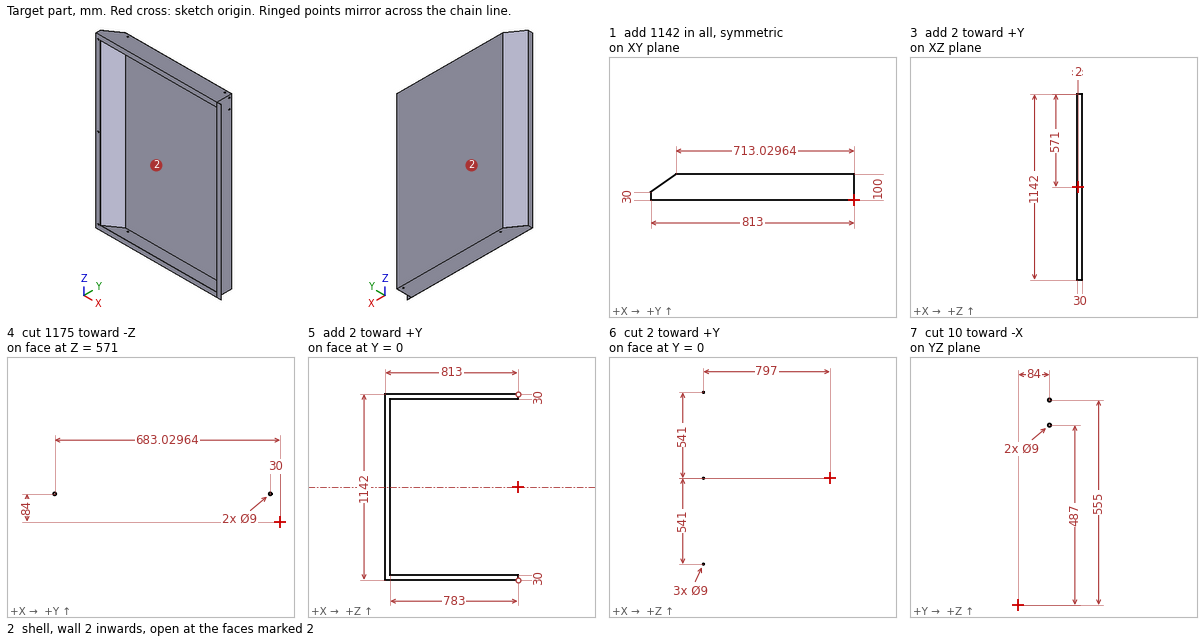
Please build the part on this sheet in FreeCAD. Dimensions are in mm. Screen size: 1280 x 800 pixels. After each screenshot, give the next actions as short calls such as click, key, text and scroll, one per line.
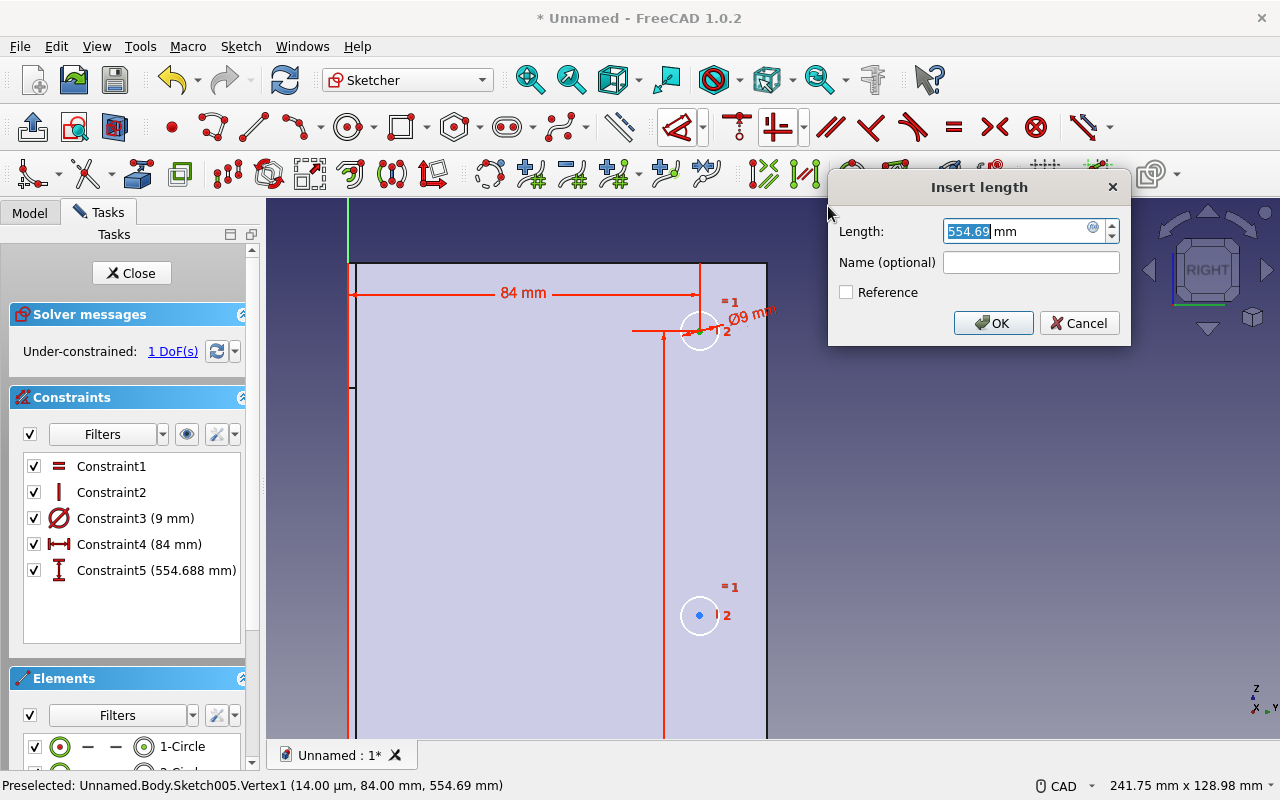
text(555)
key(Return)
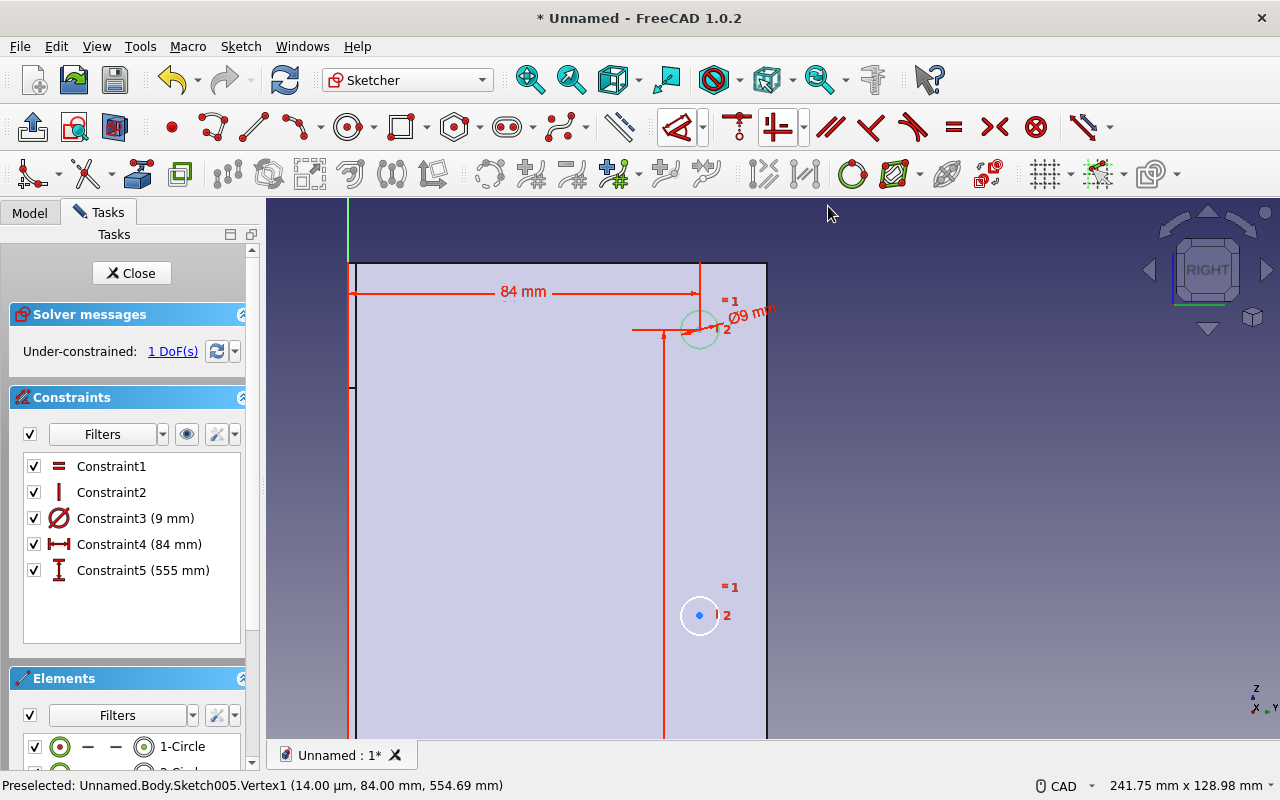
click(700, 616)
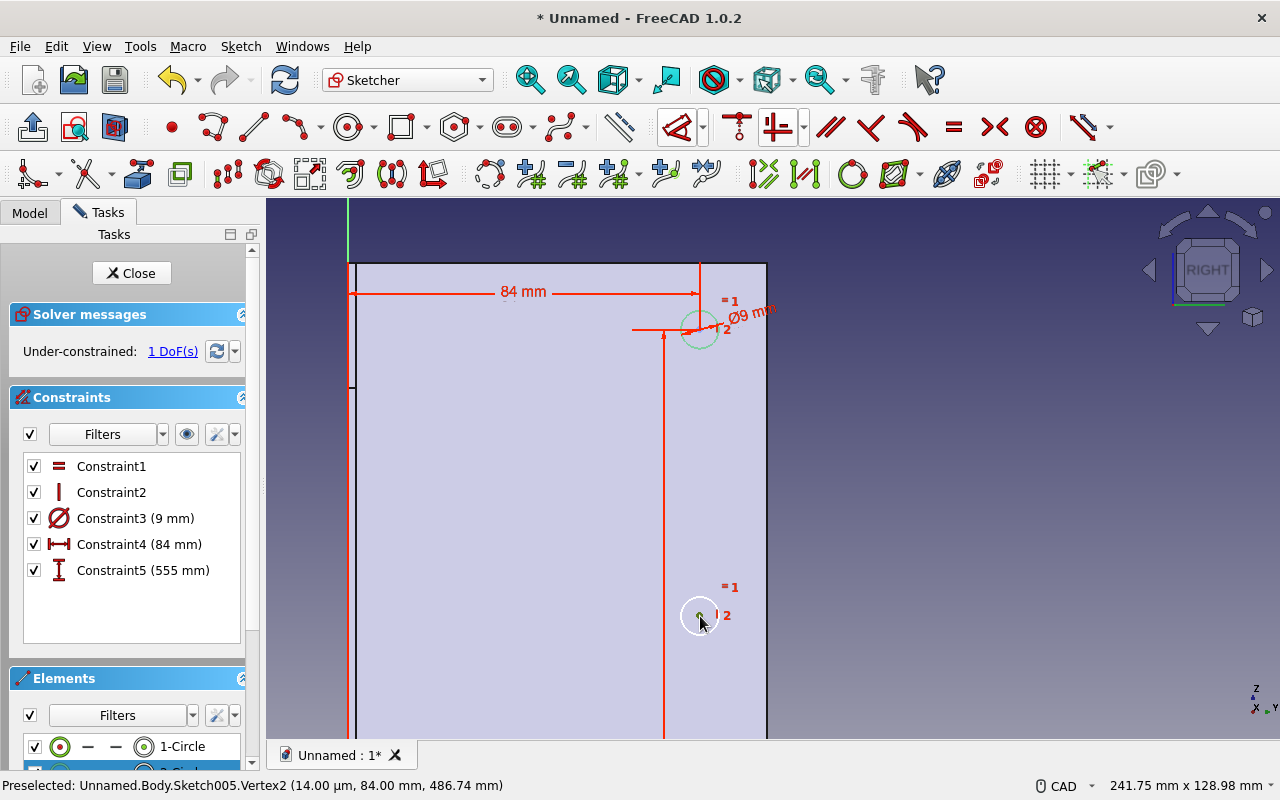
key(i)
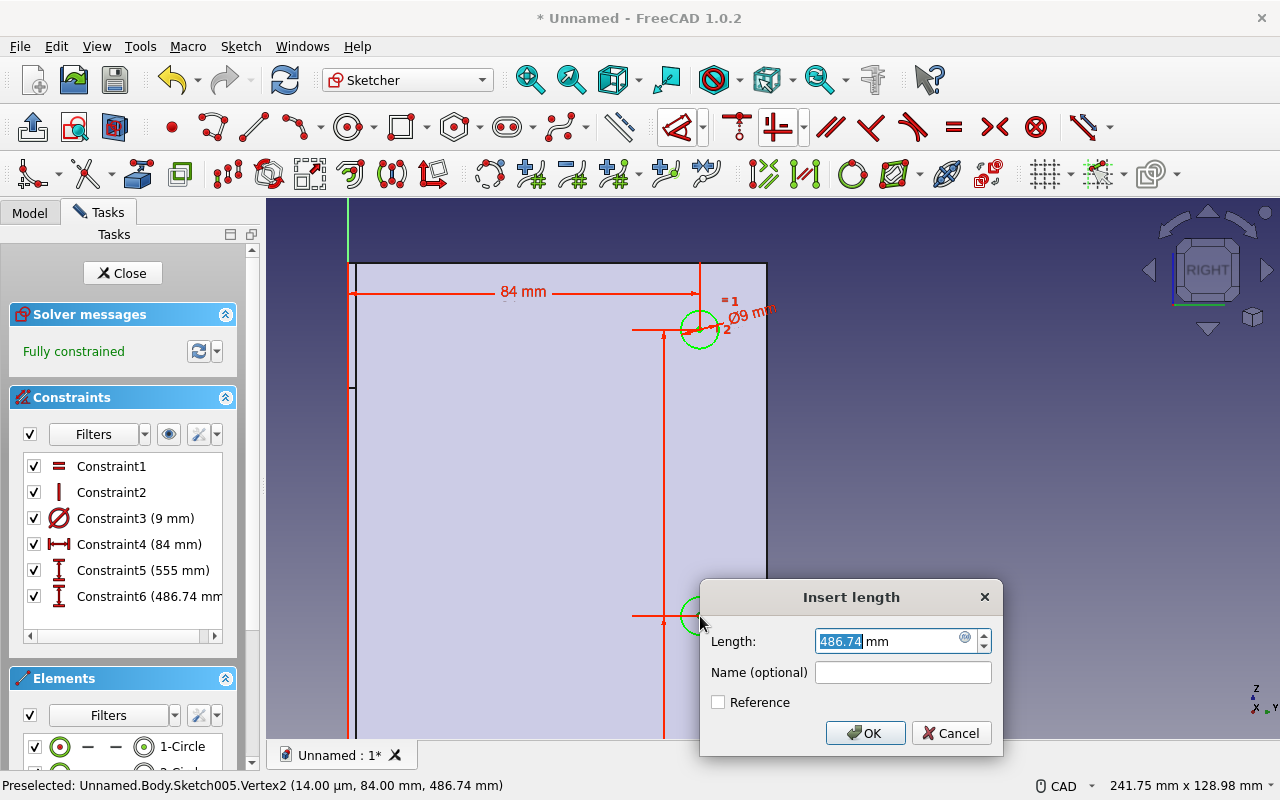
text(487)
key(Return)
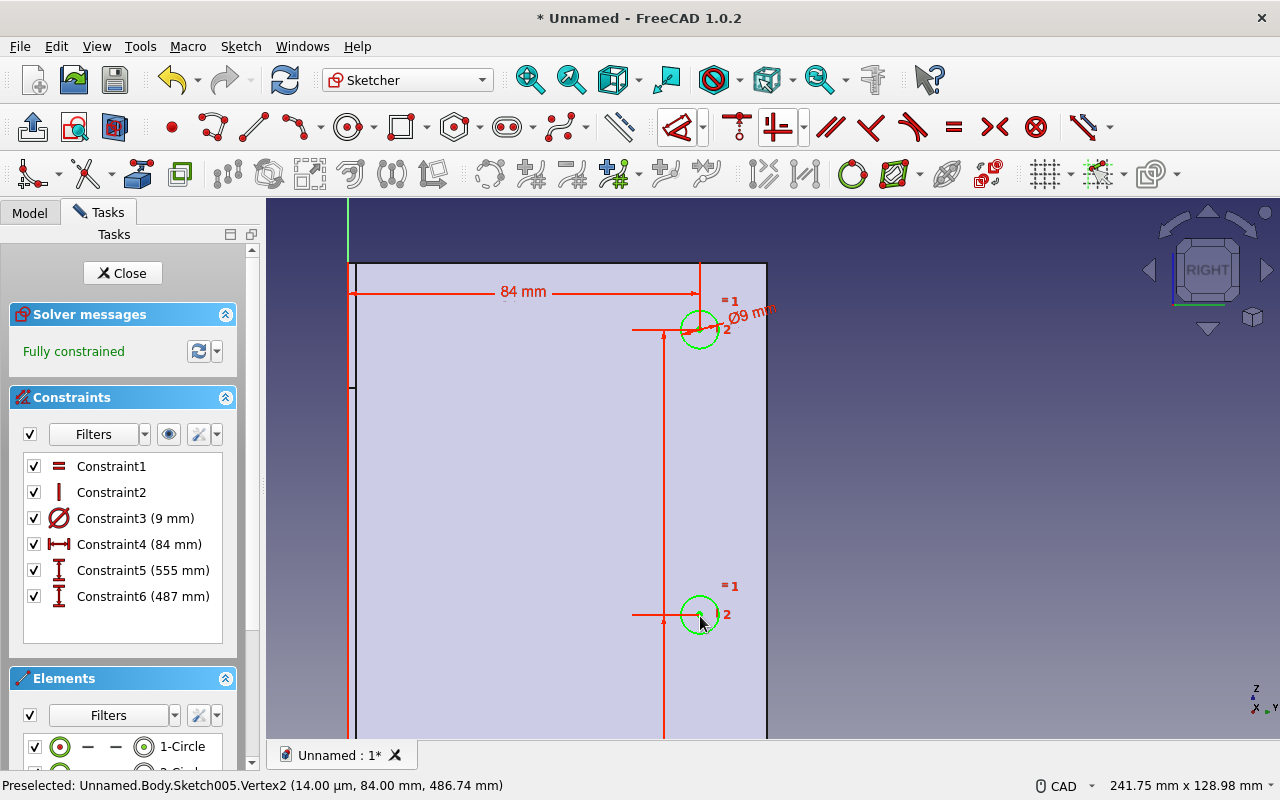
click(123, 273)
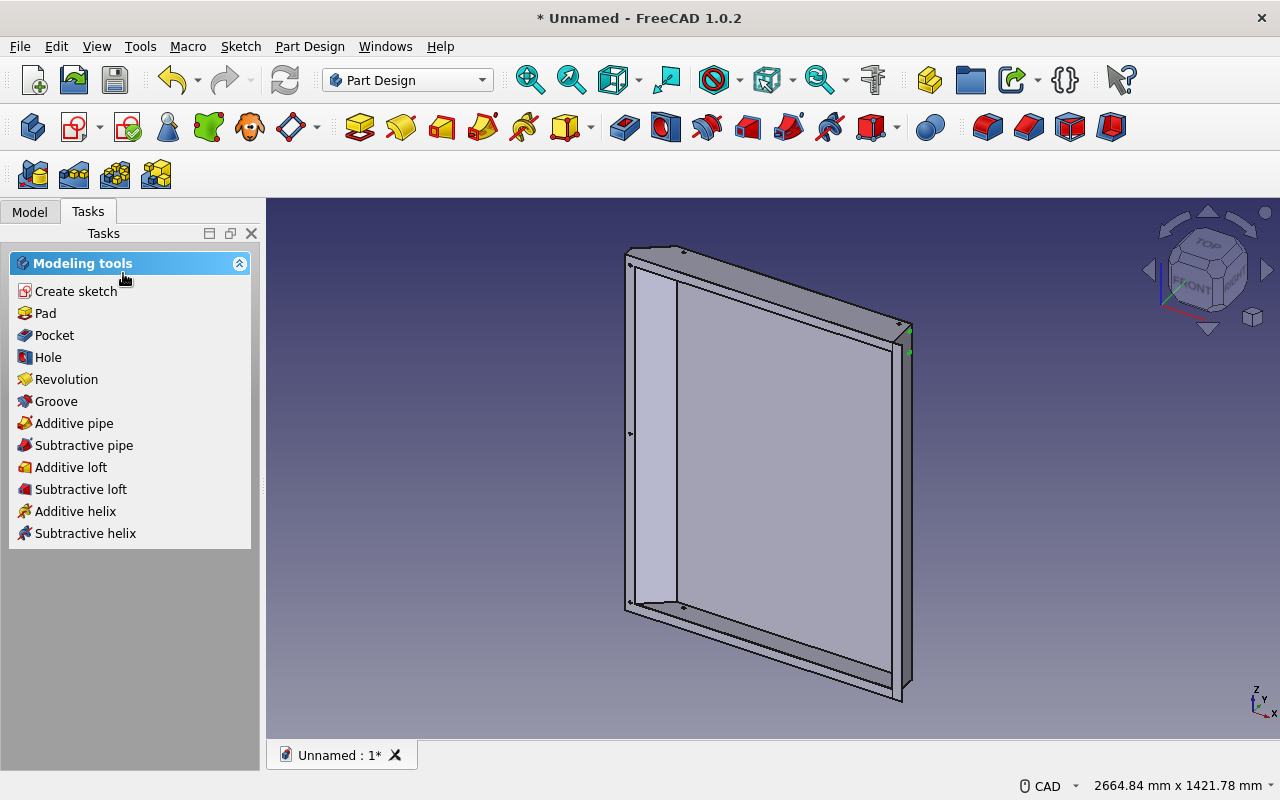
click(625, 128)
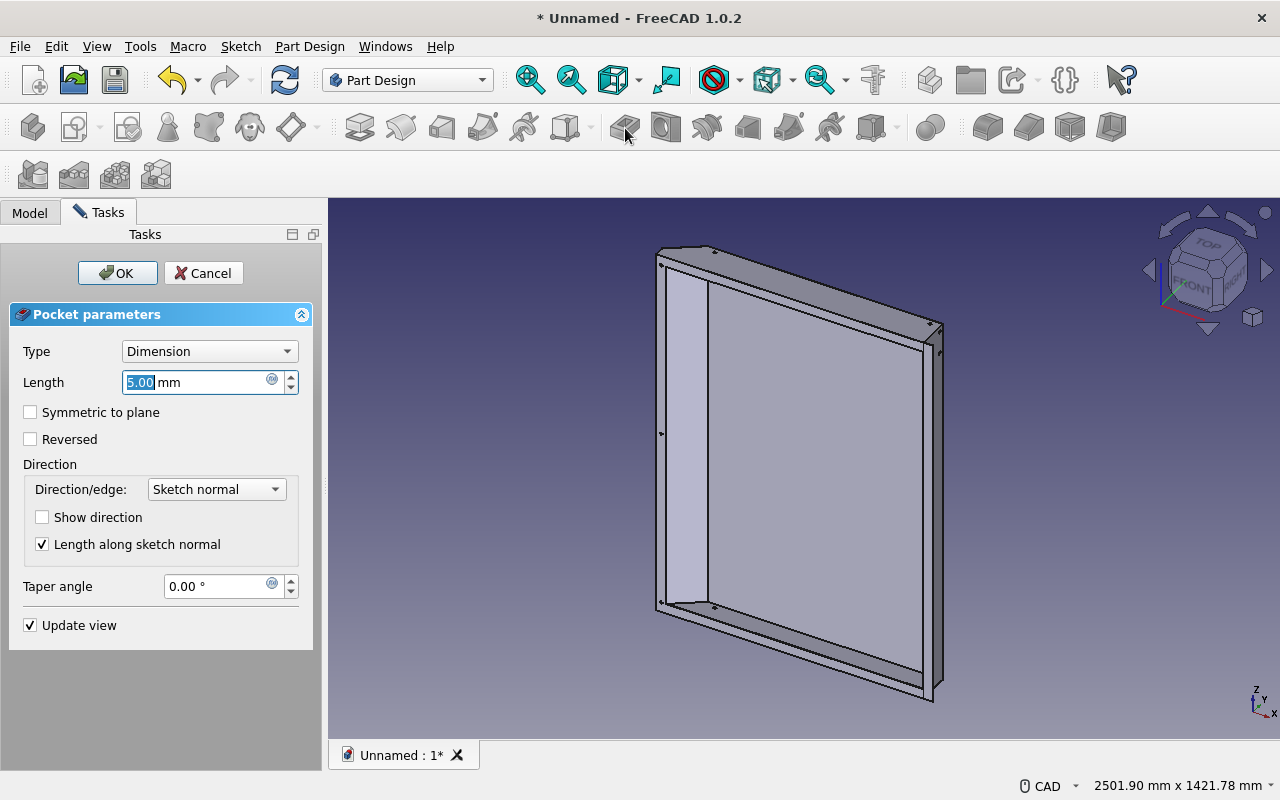
text(10)
key(Tab)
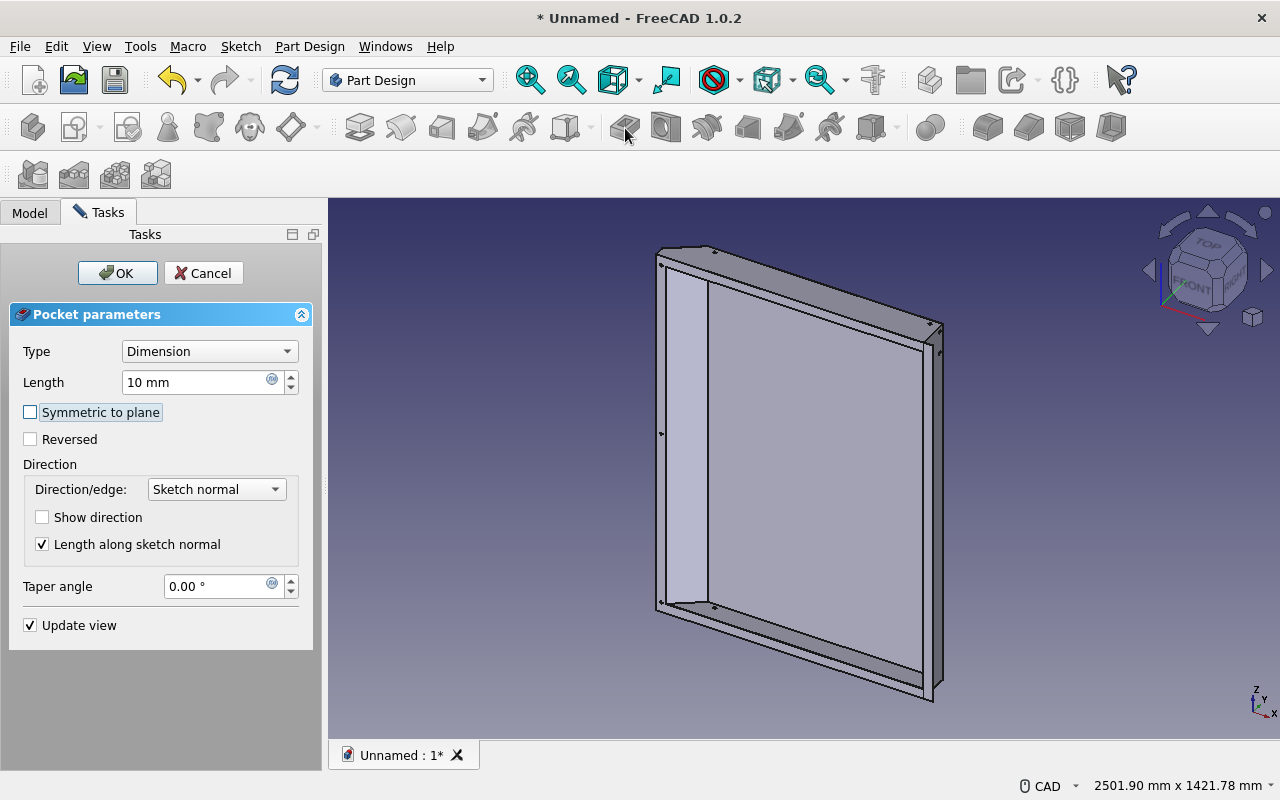
click(118, 273)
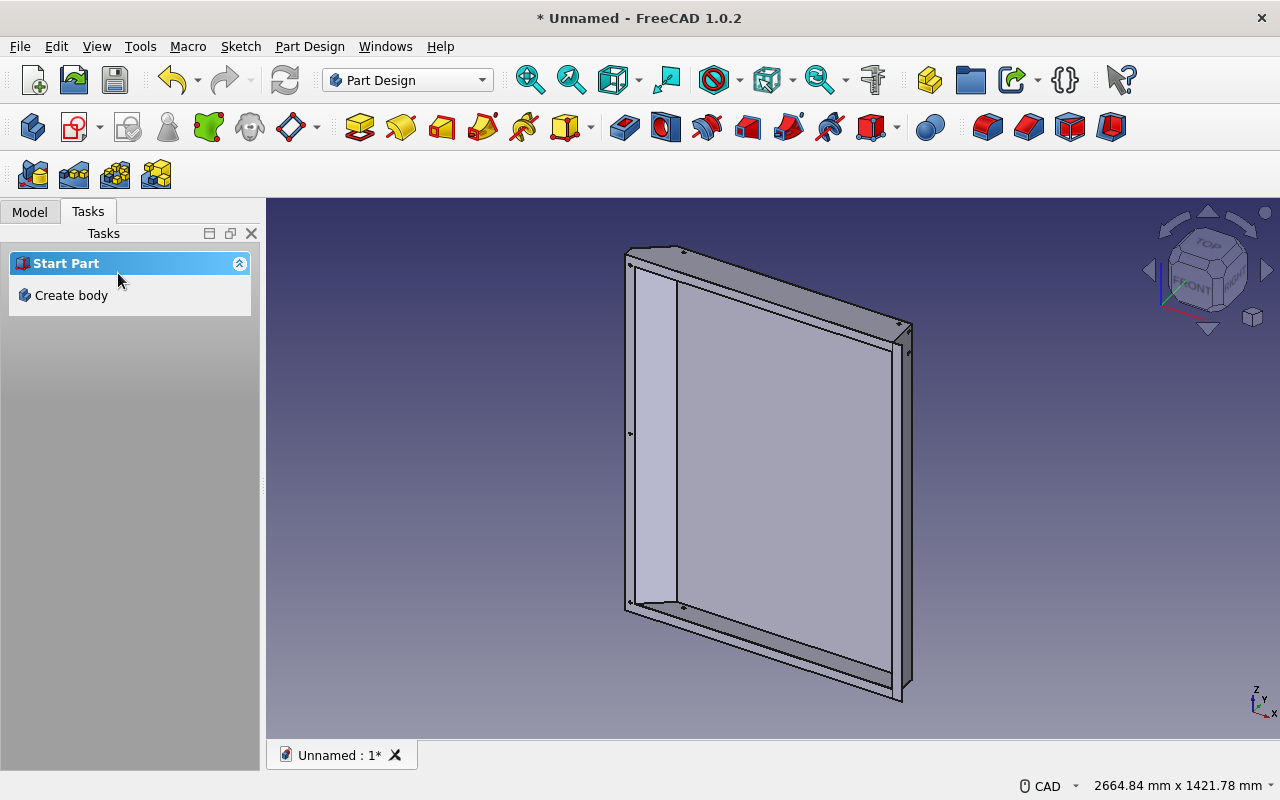
key(0)